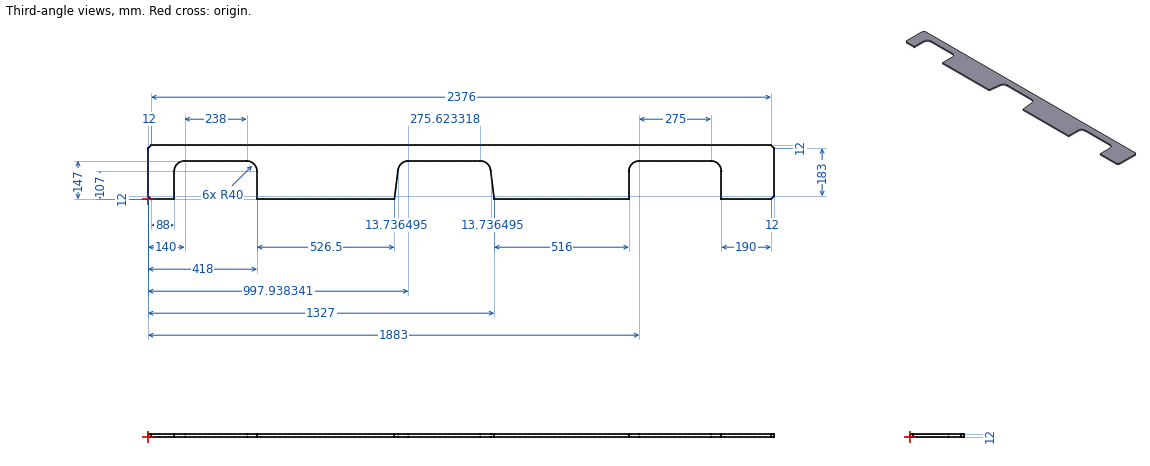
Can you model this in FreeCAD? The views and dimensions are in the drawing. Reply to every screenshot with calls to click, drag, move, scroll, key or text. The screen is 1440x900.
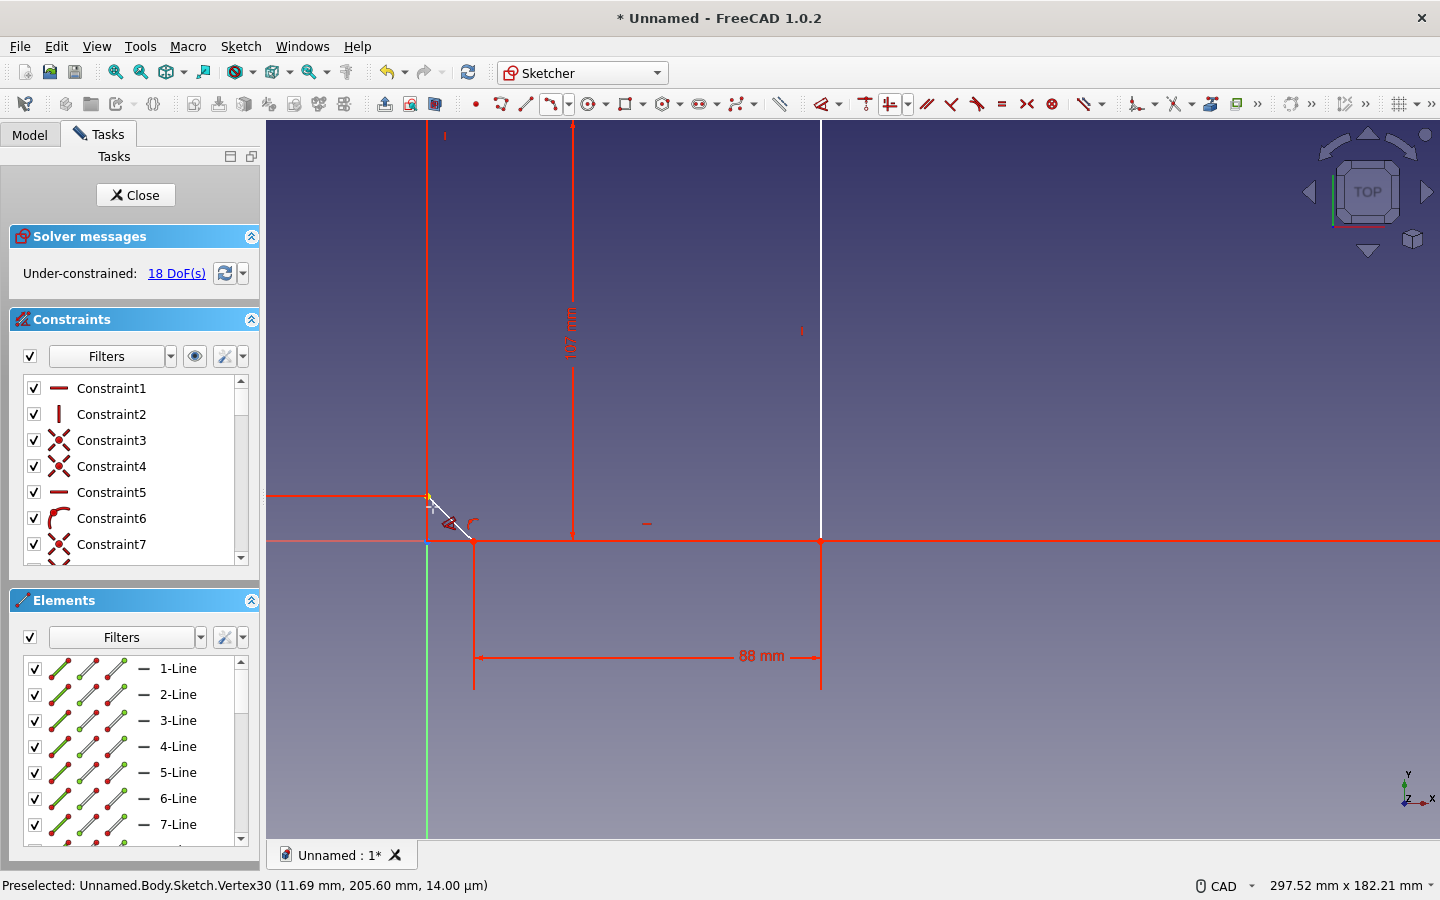
click(427, 496)
click(393, 519)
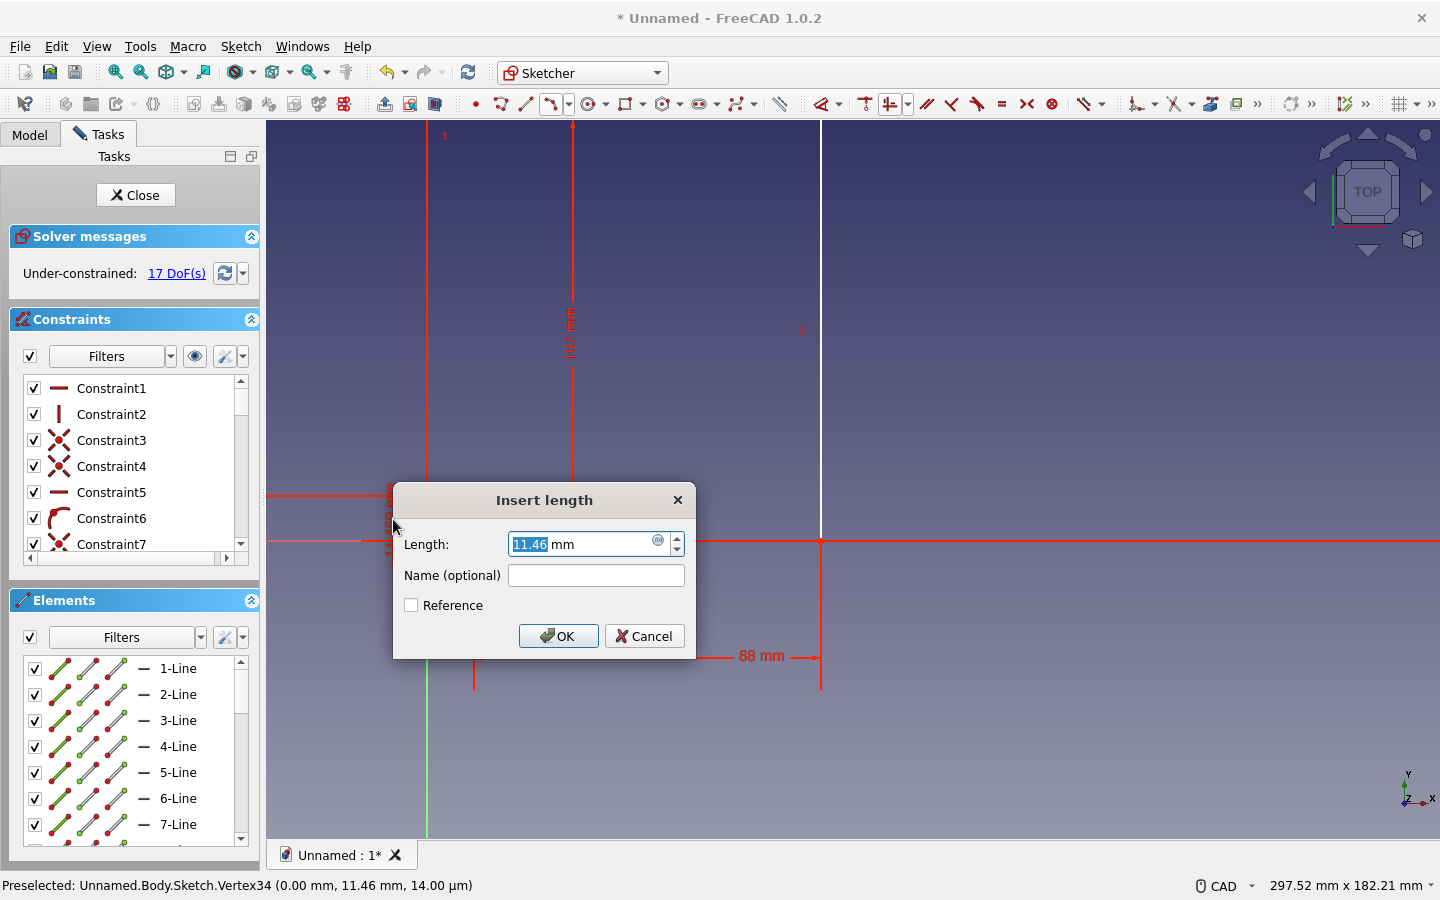
text(12)
key(Return)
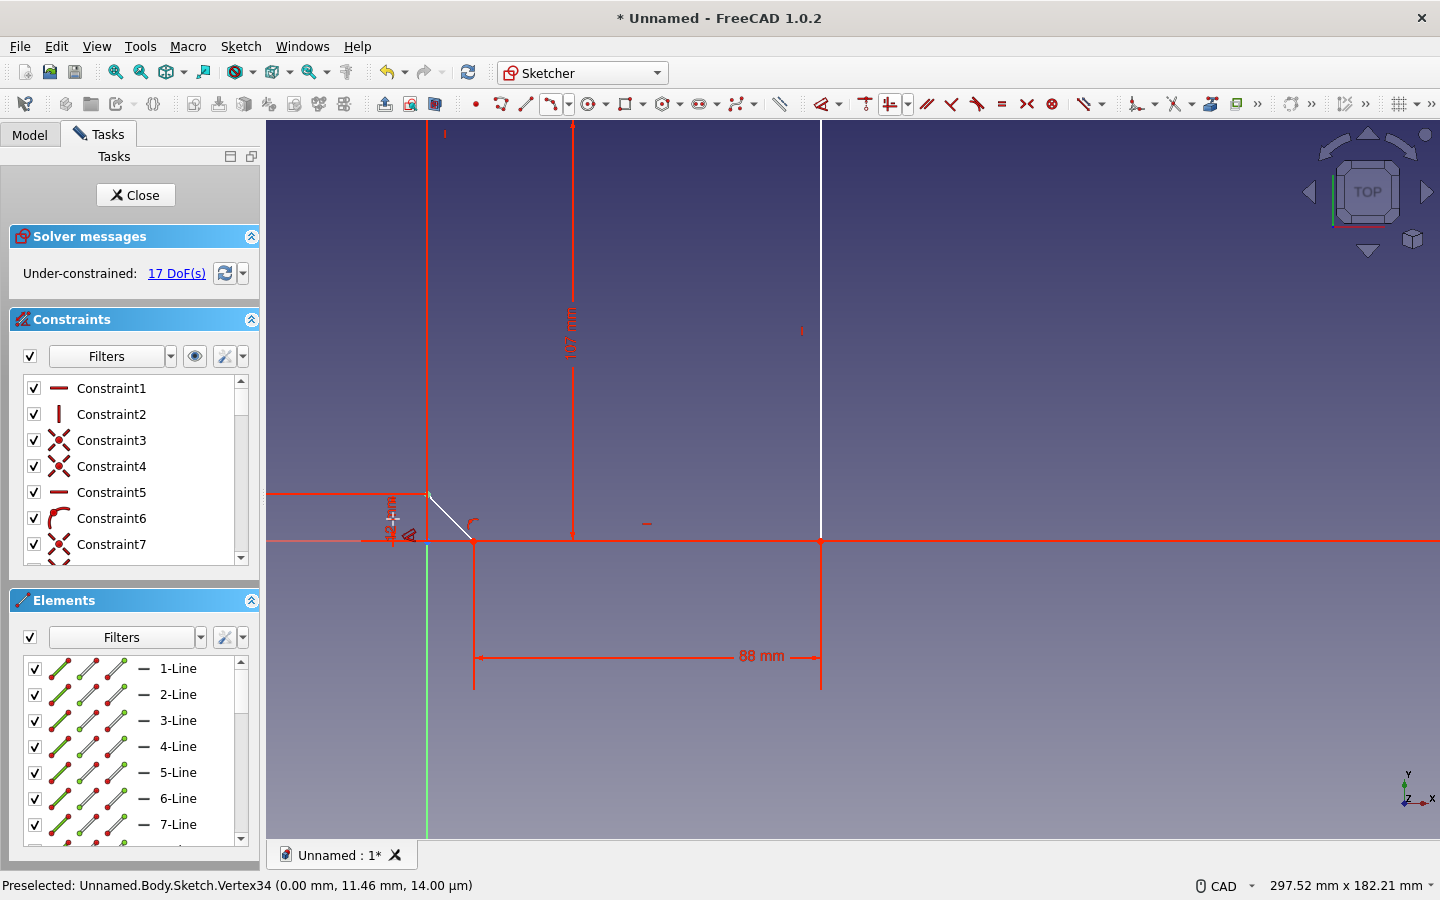
click(474, 541)
click(450, 575)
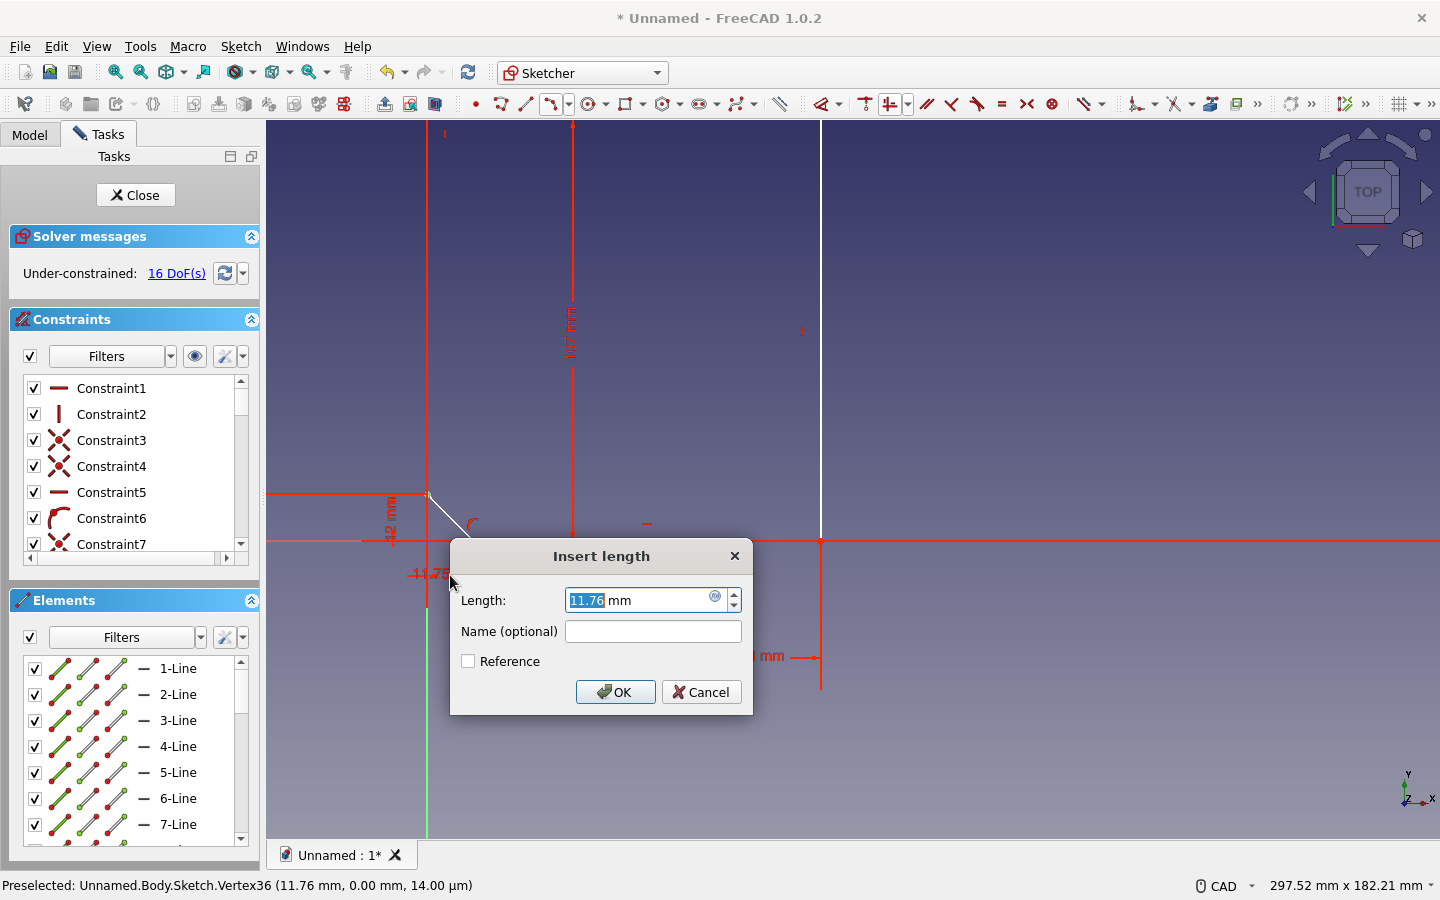
text(12)
key(Return)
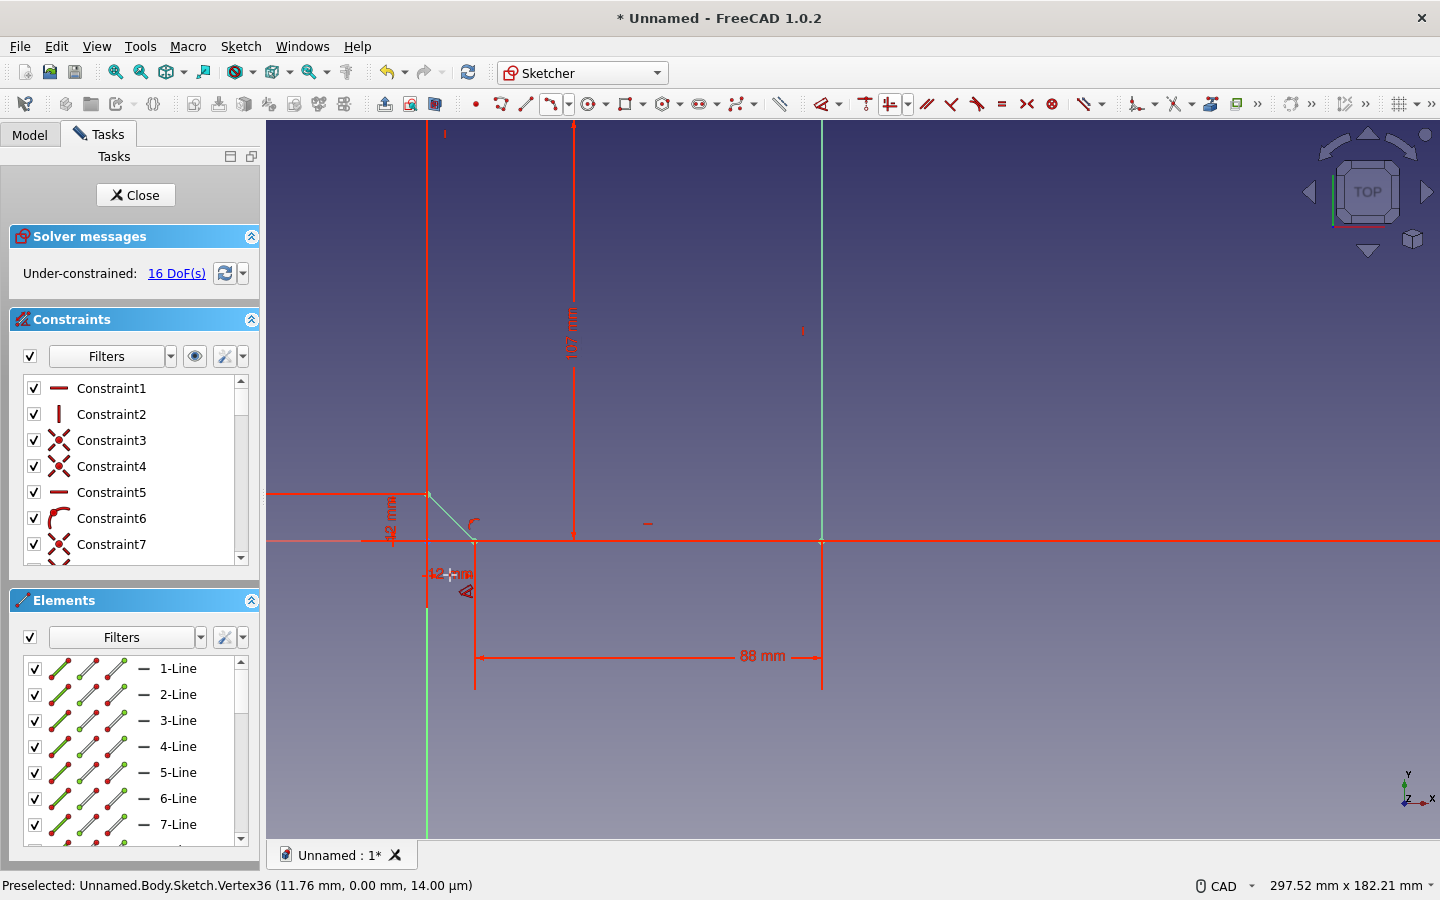
scroll(433, 507, down, 13)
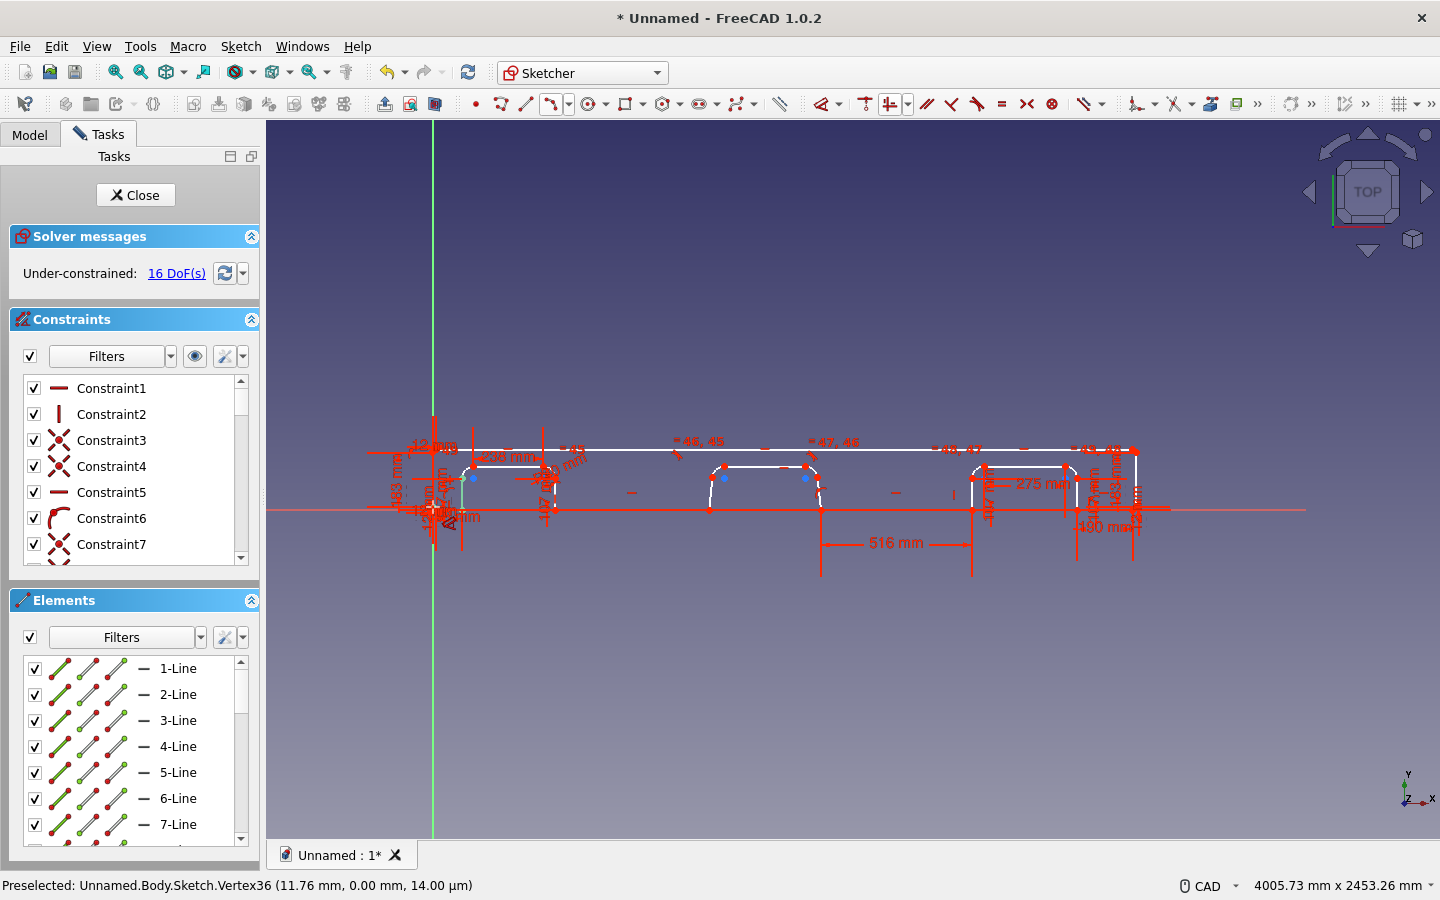
scroll(1134, 509, up, 13)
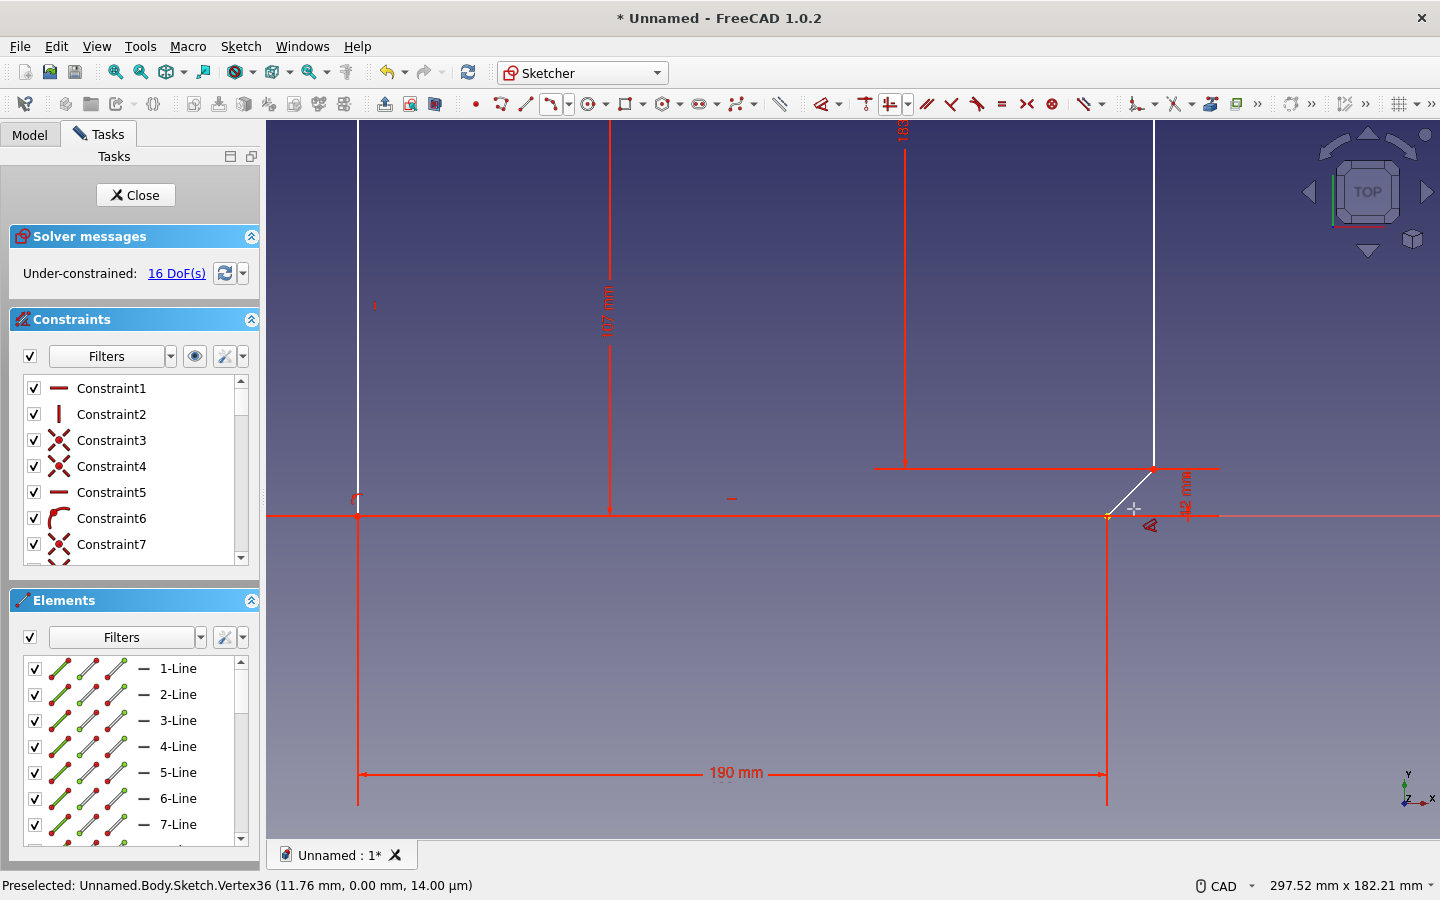
click(1121, 502)
click(1131, 550)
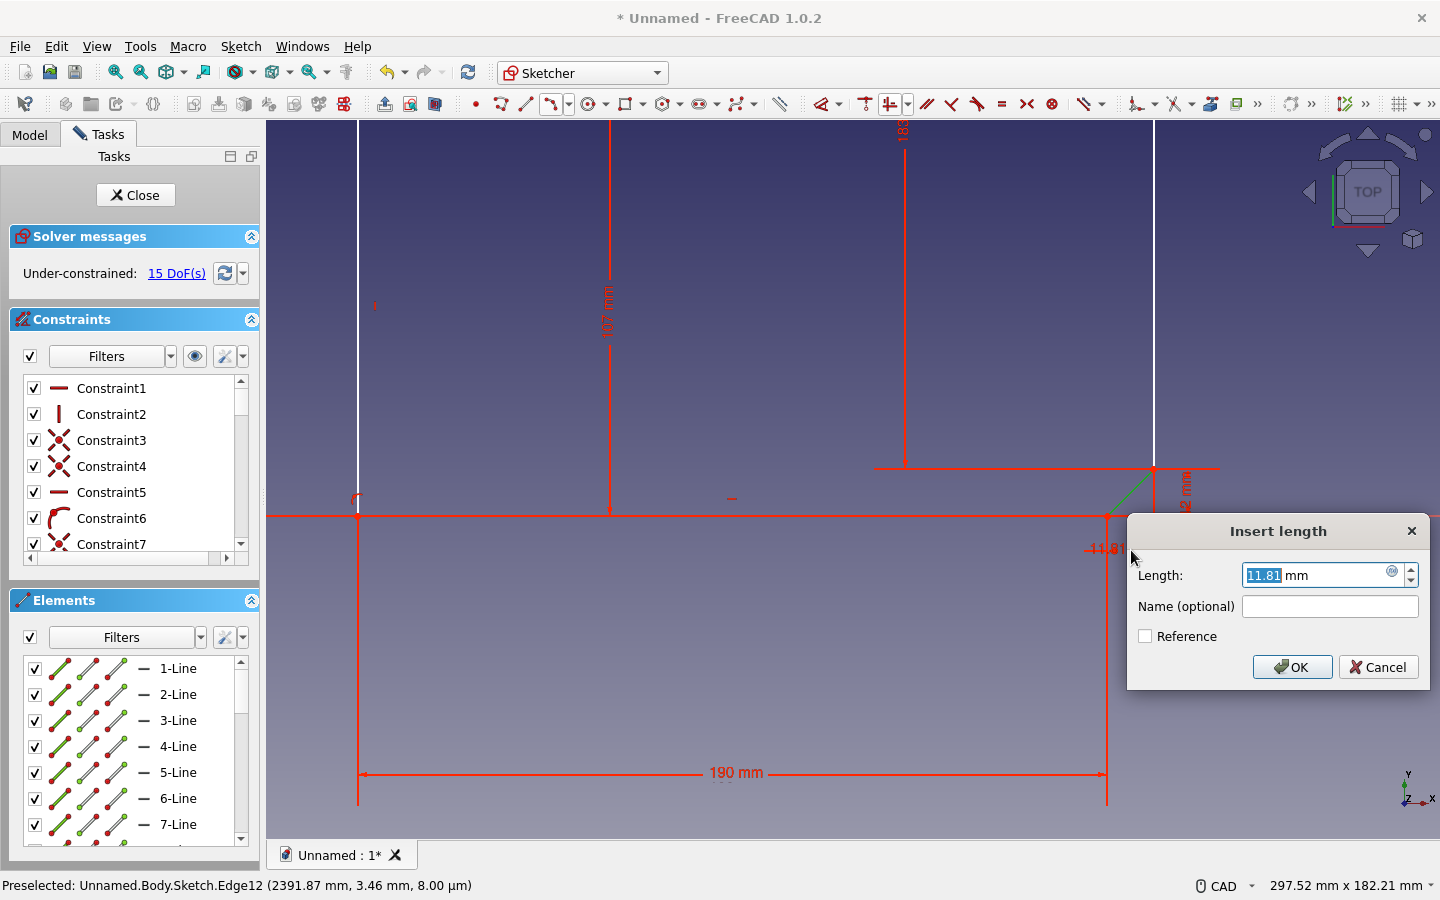
text(12)
key(Return)